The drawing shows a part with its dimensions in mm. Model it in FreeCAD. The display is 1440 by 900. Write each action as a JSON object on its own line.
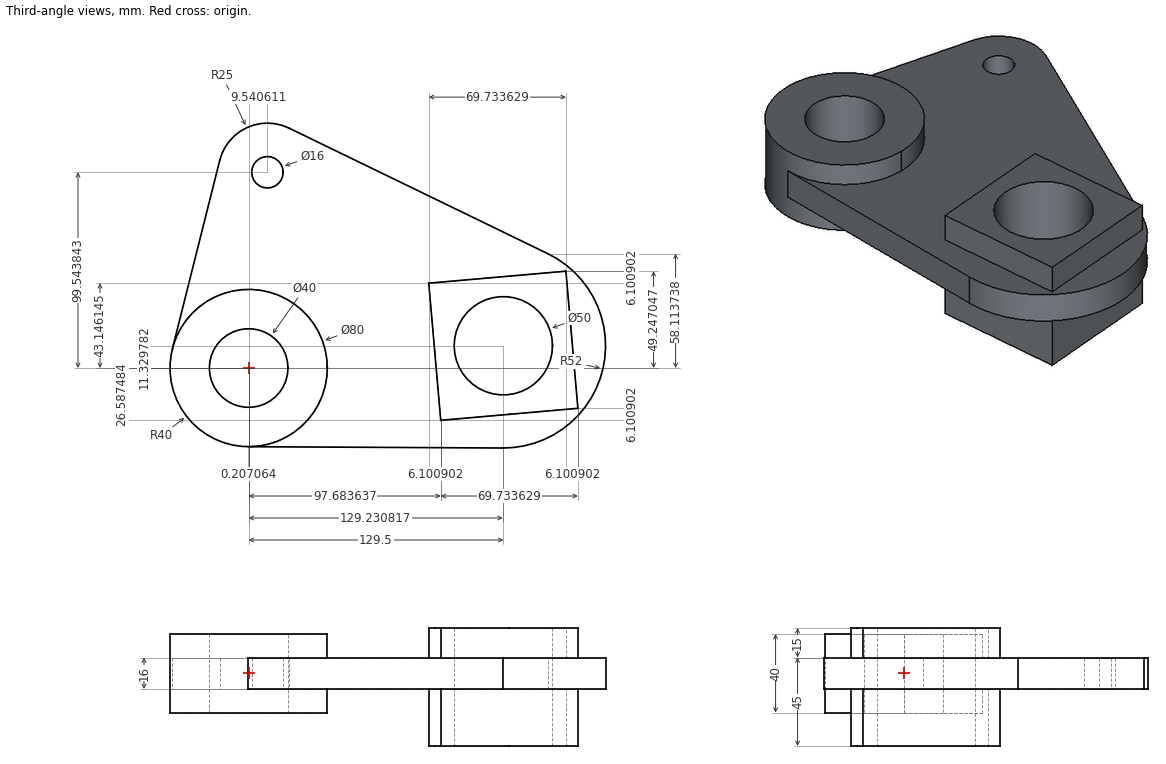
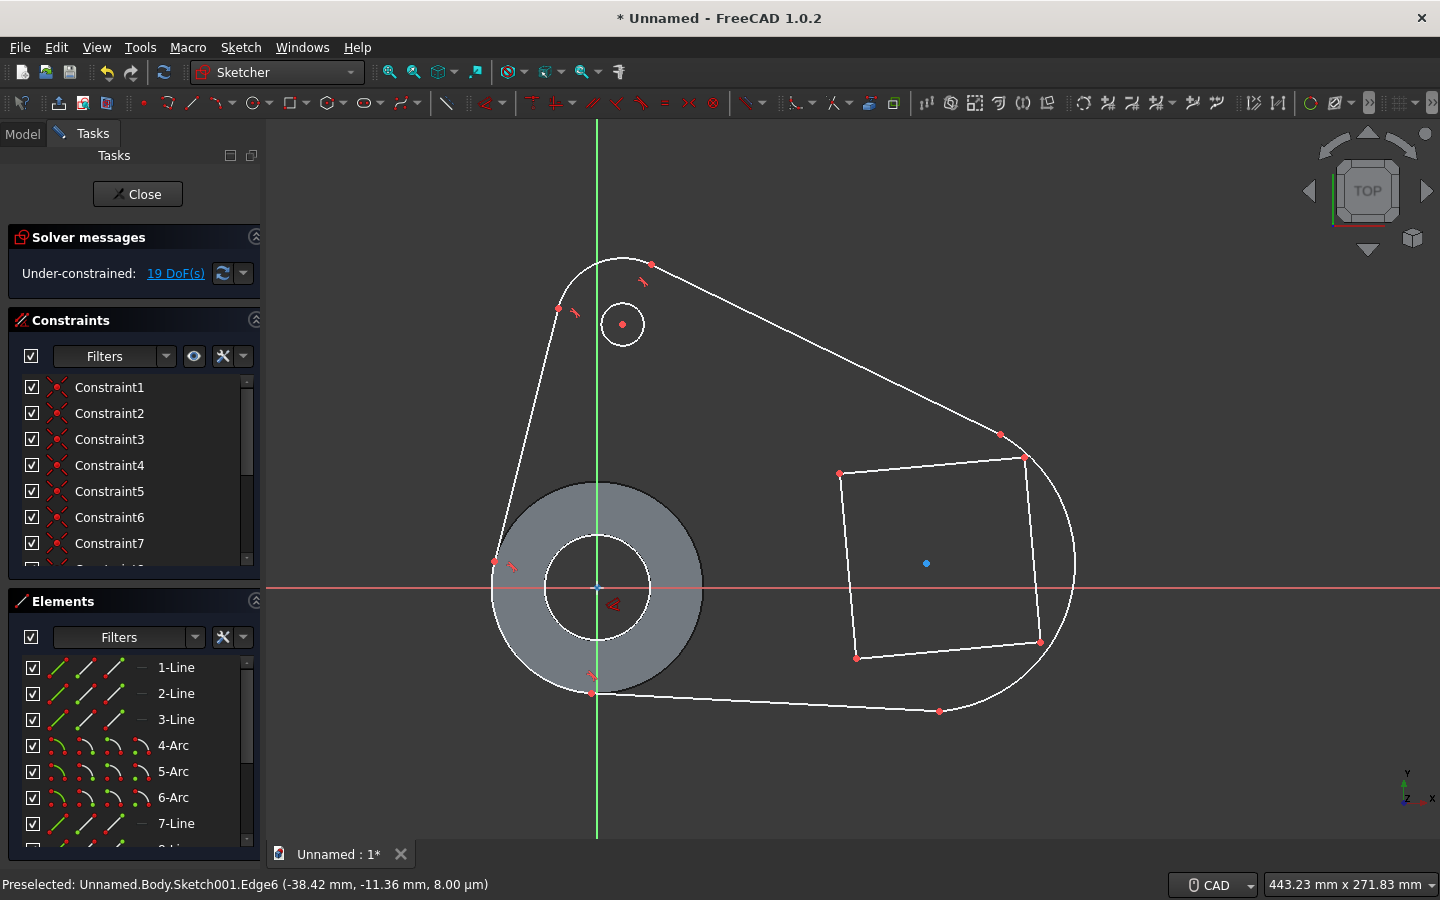
{"action": "left_click", "coordinate": [1038, 662]}
{"action": "left_click", "coordinate": [1062, 683]}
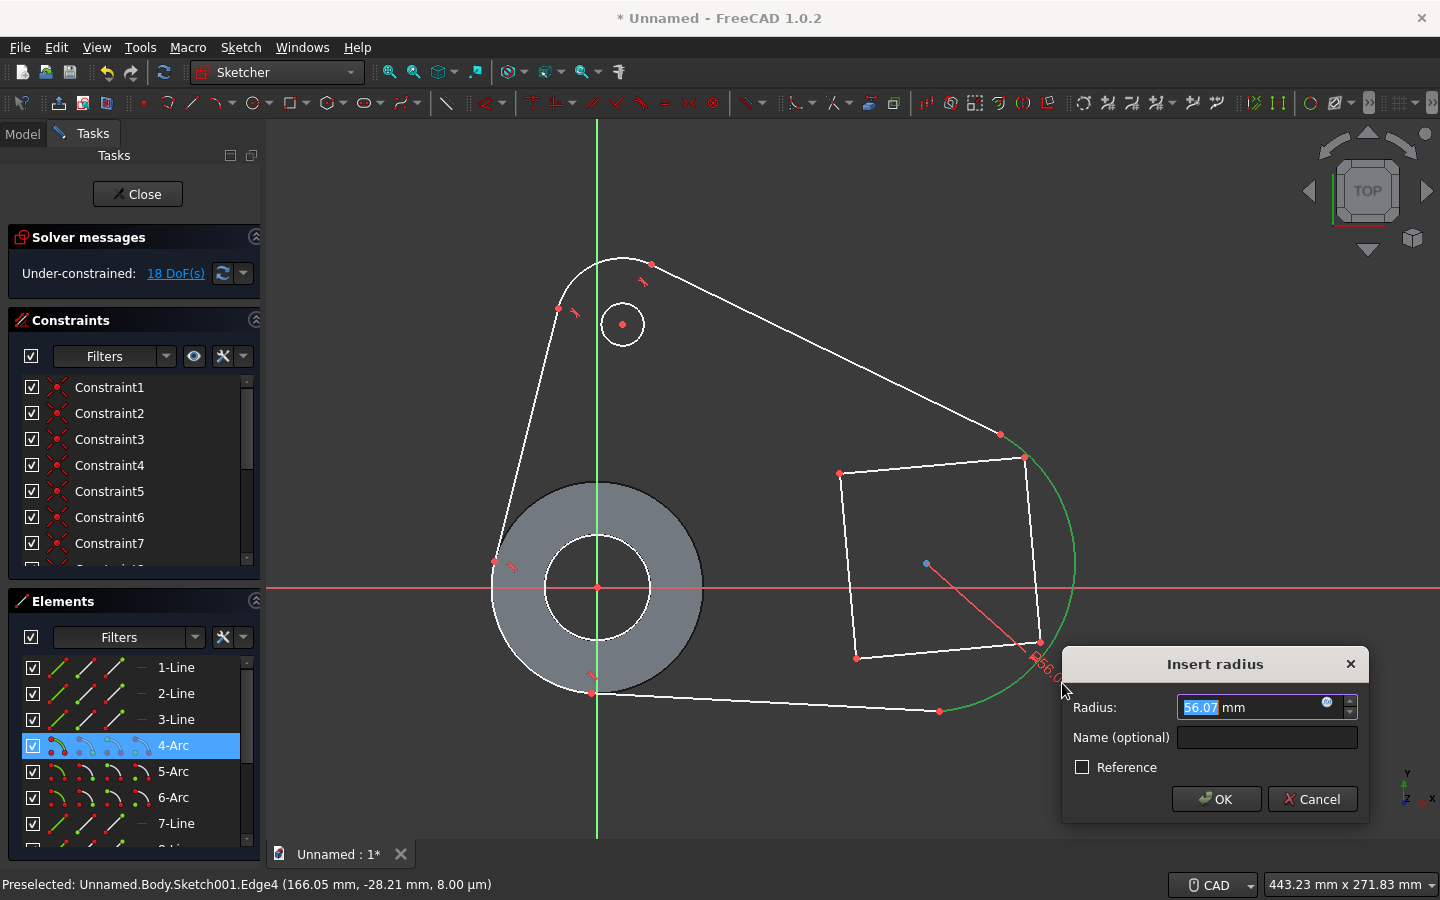
{"action": "type", "text": "52"}
{"action": "key", "text": "Return"}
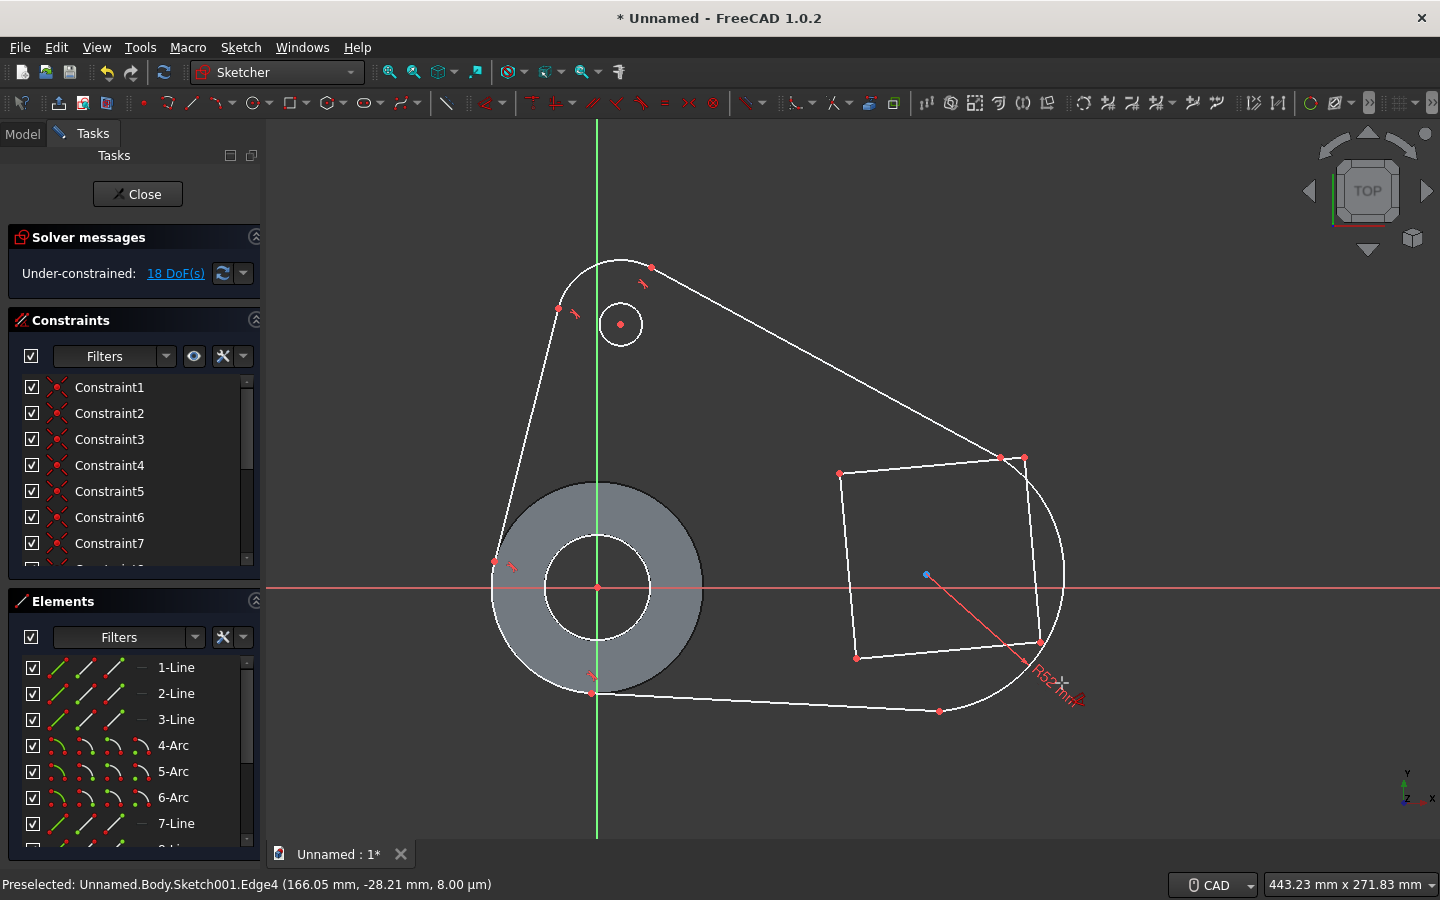
{"action": "left_click", "coordinate": [618, 260]}
{"action": "left_click", "coordinate": [617, 228]}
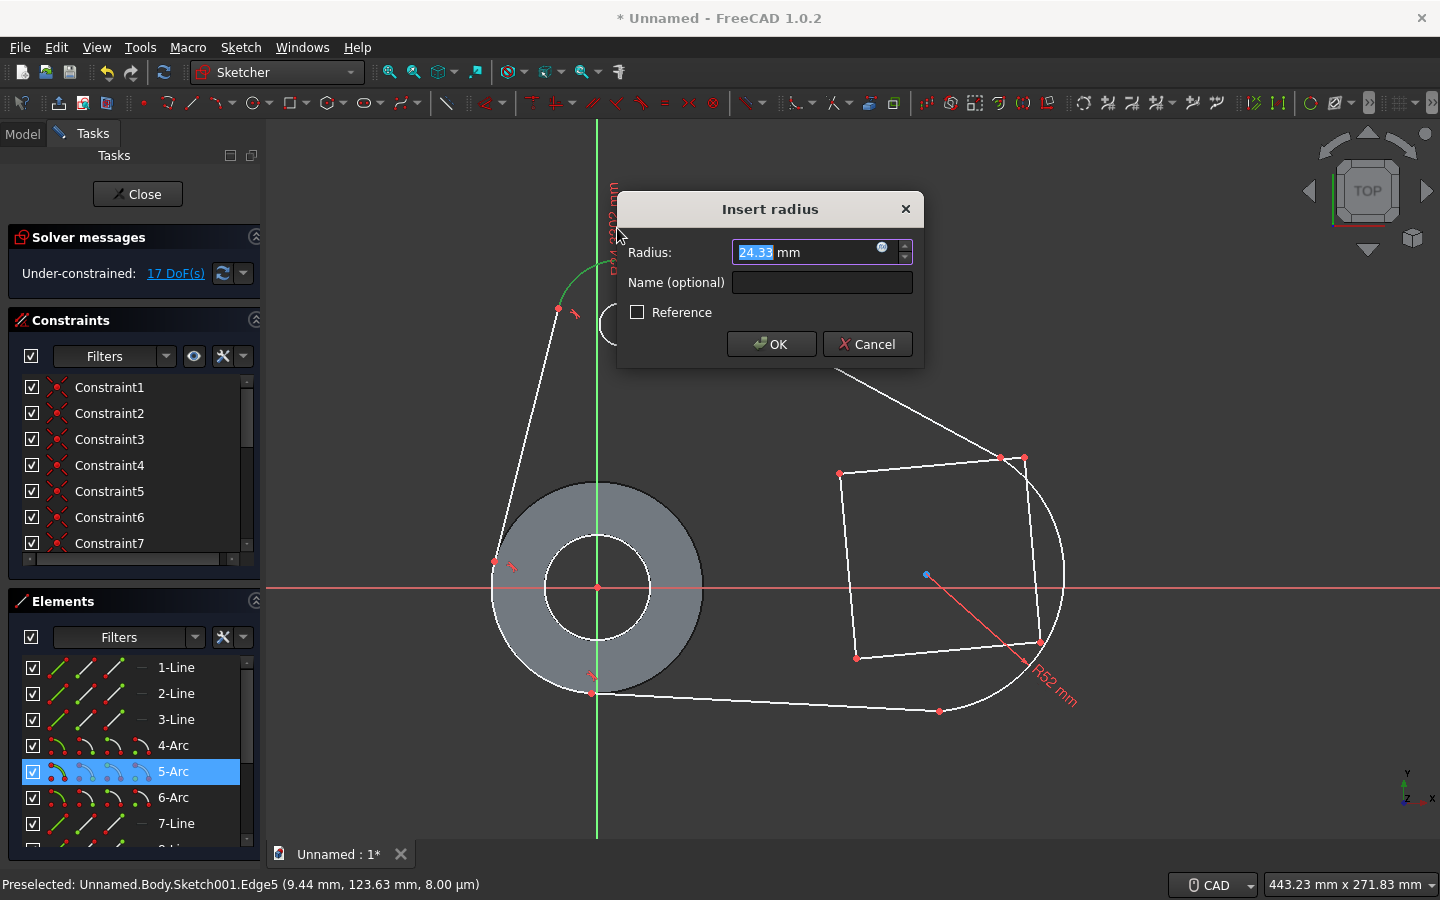
{"action": "type", "text": "25"}
{"action": "key", "text": "Return"}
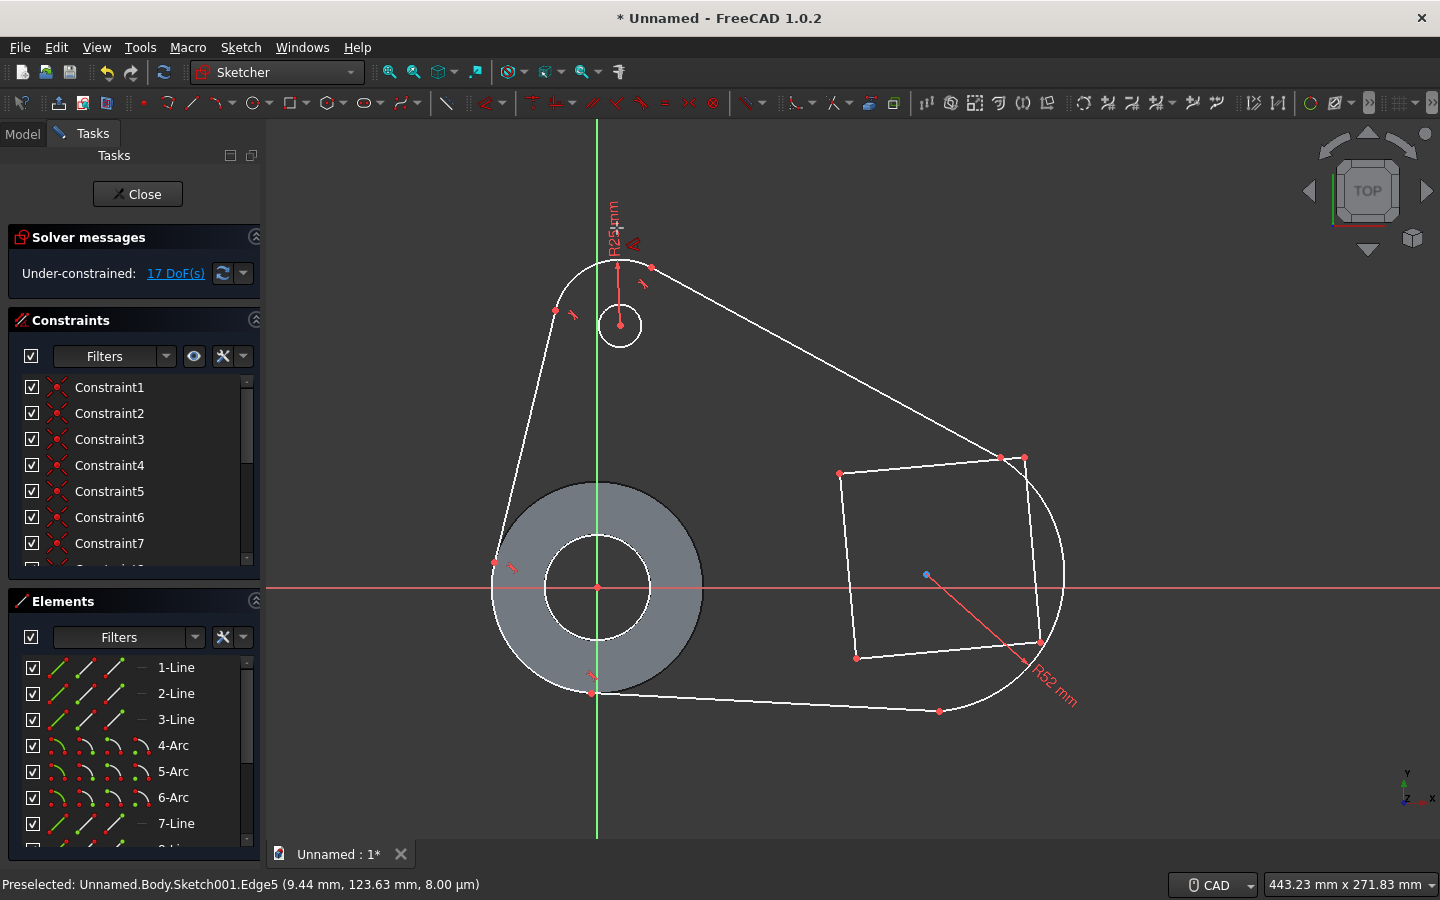
{"action": "left_click", "coordinate": [496, 618]}
{"action": "left_click", "coordinate": [465, 627]}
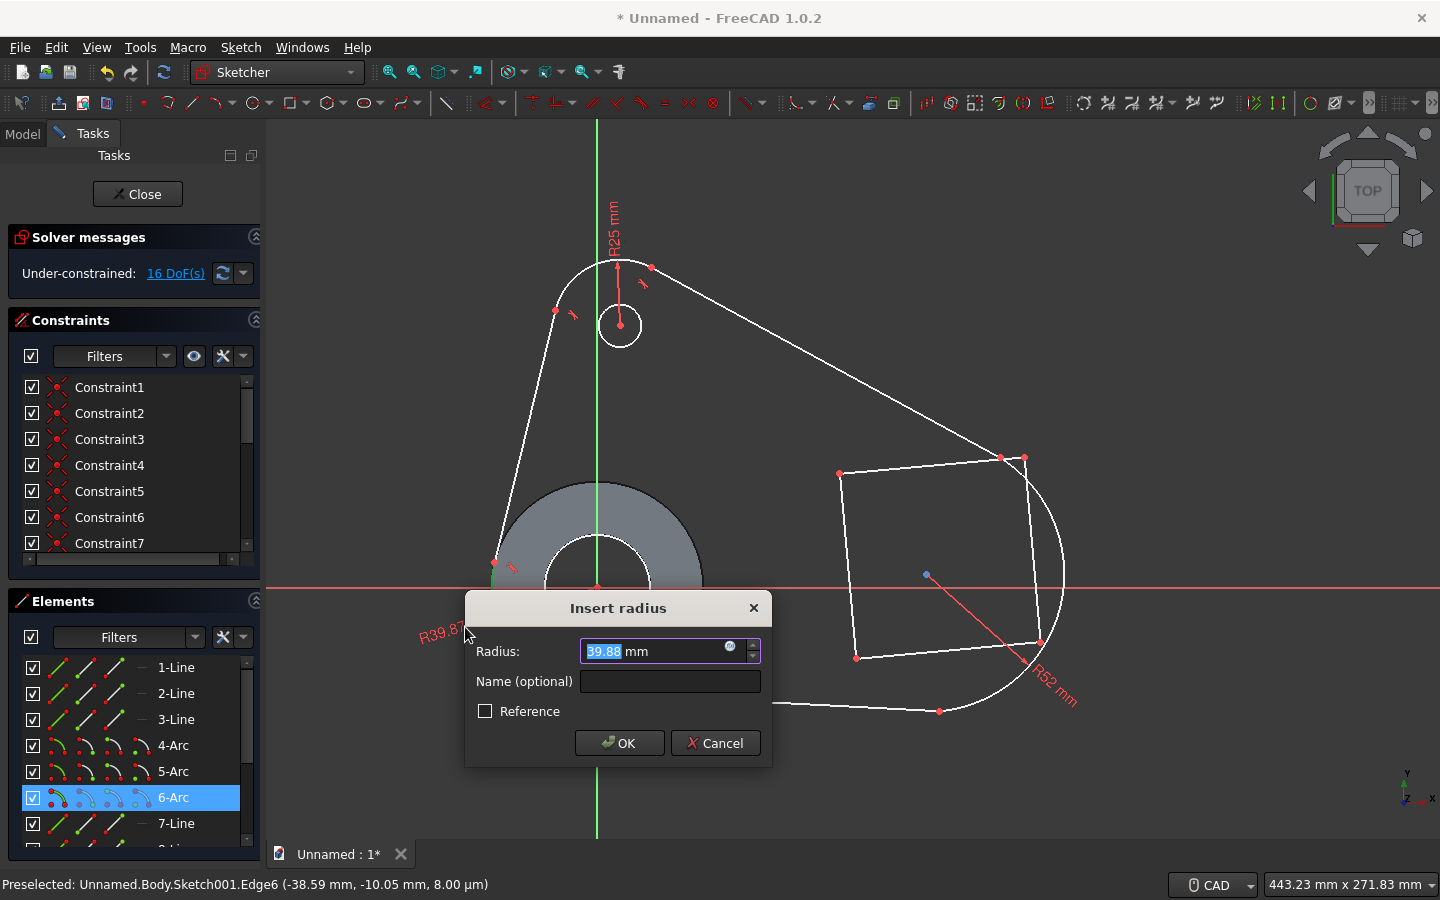
{"action": "type", "text": "40"}
{"action": "key", "text": "Return"}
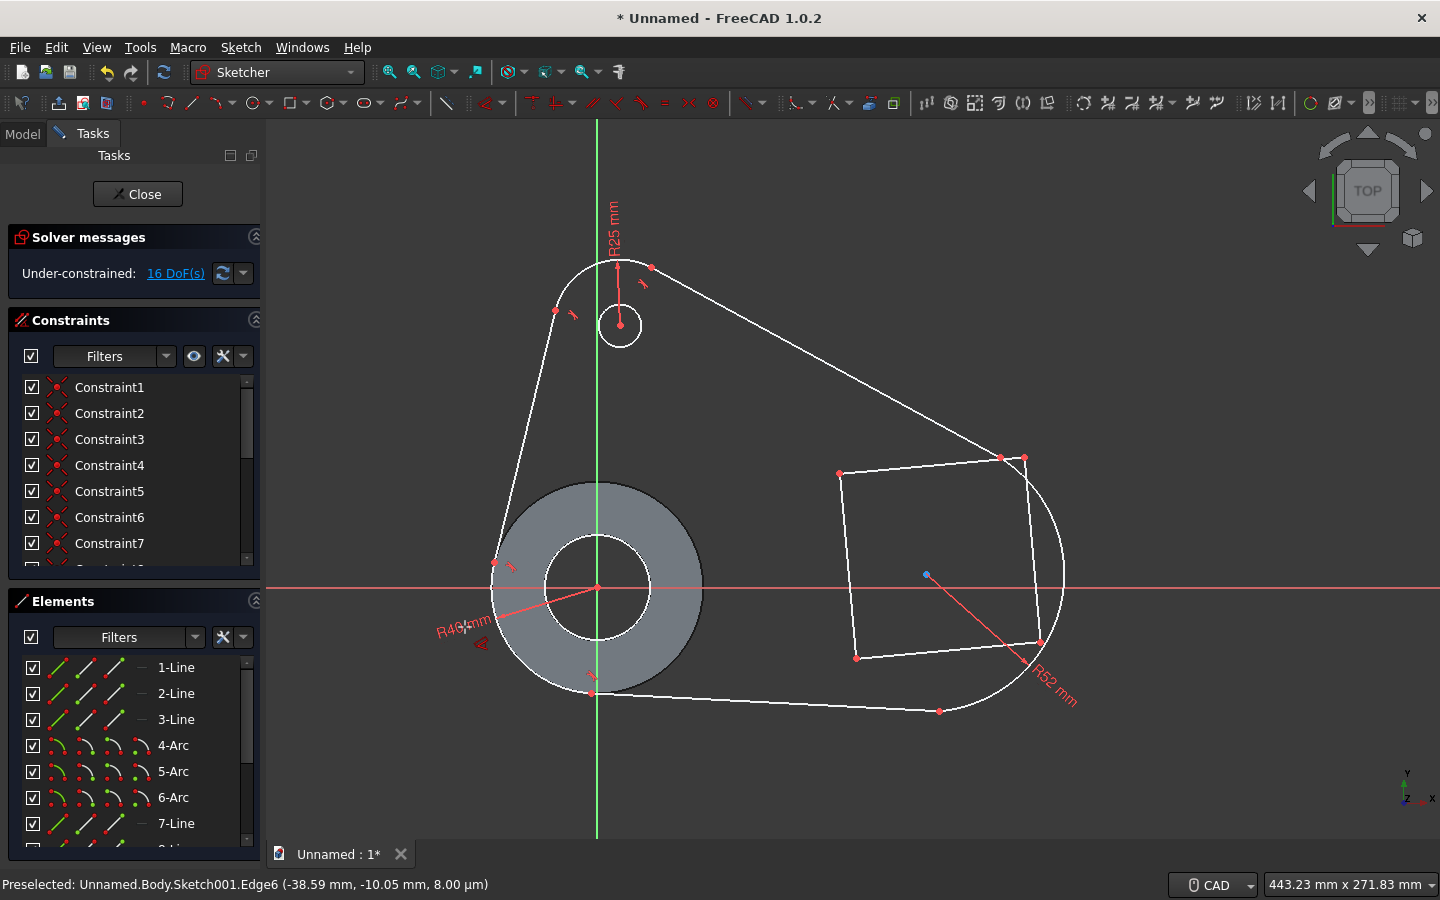
{"action": "left_click", "coordinate": [634, 550]}
{"action": "left_click", "coordinate": [656, 527]}